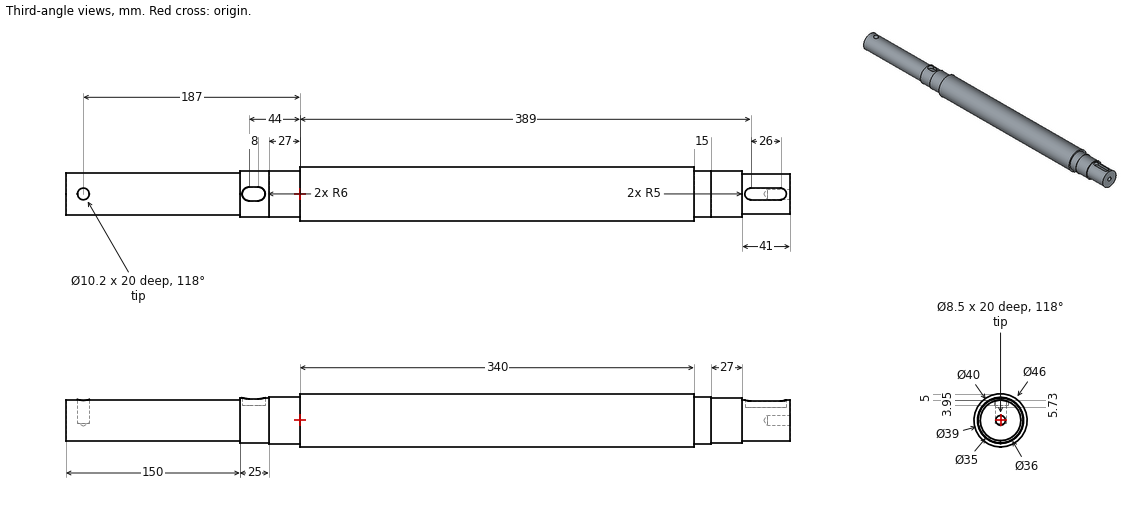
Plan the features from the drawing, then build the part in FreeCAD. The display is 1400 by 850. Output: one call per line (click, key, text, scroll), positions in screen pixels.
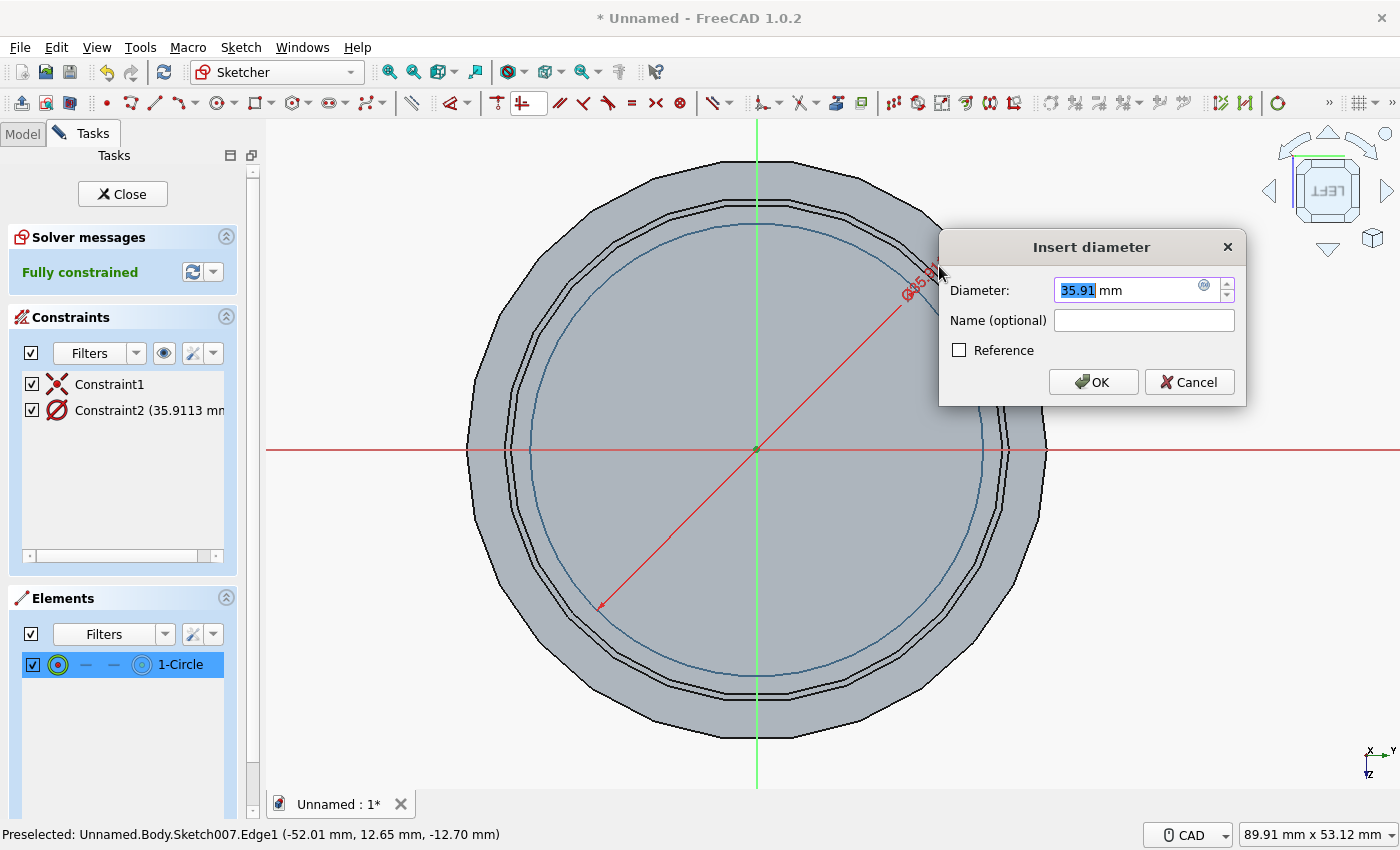
text(36)
key(Return)
key(Escape)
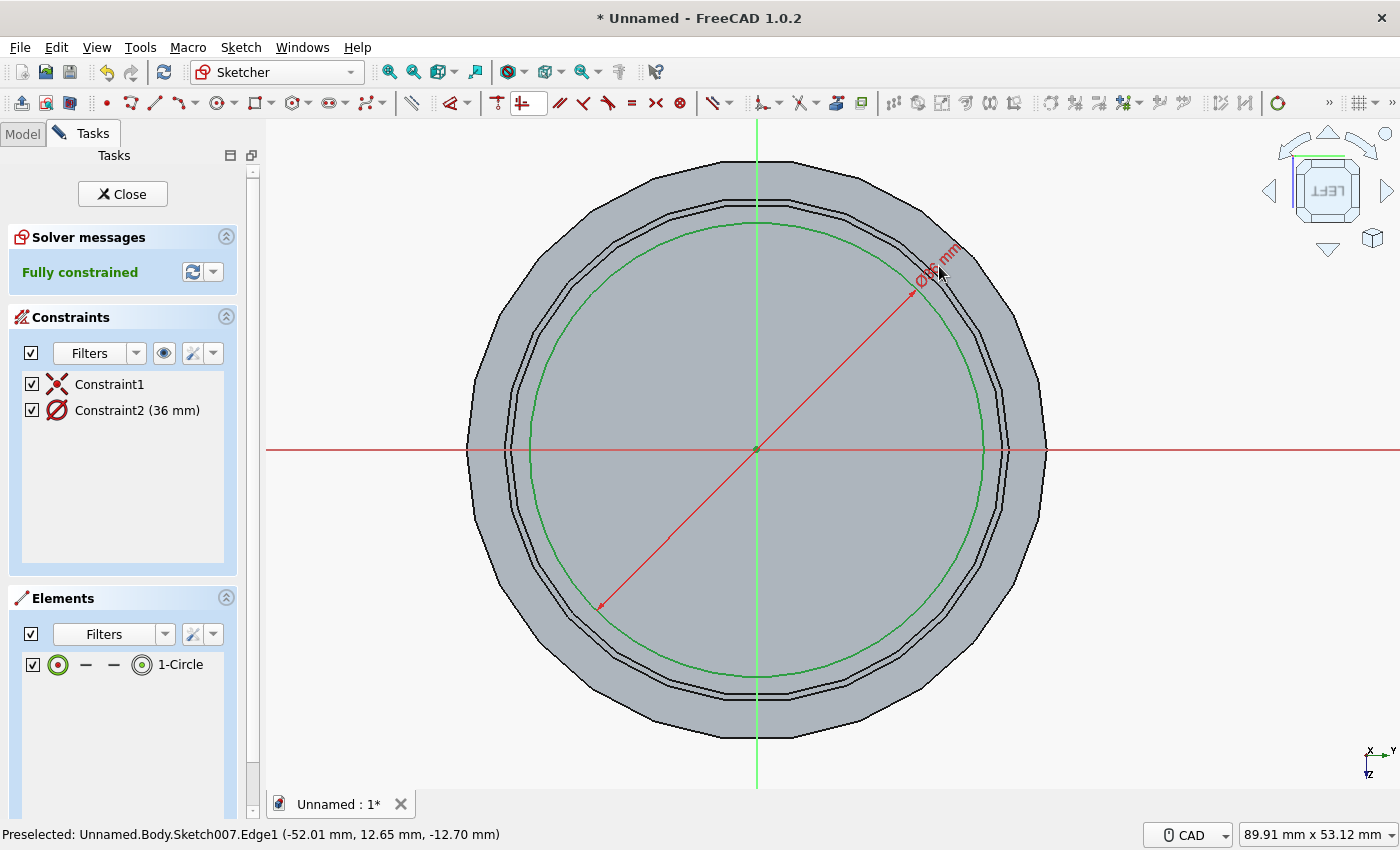
click(123, 194)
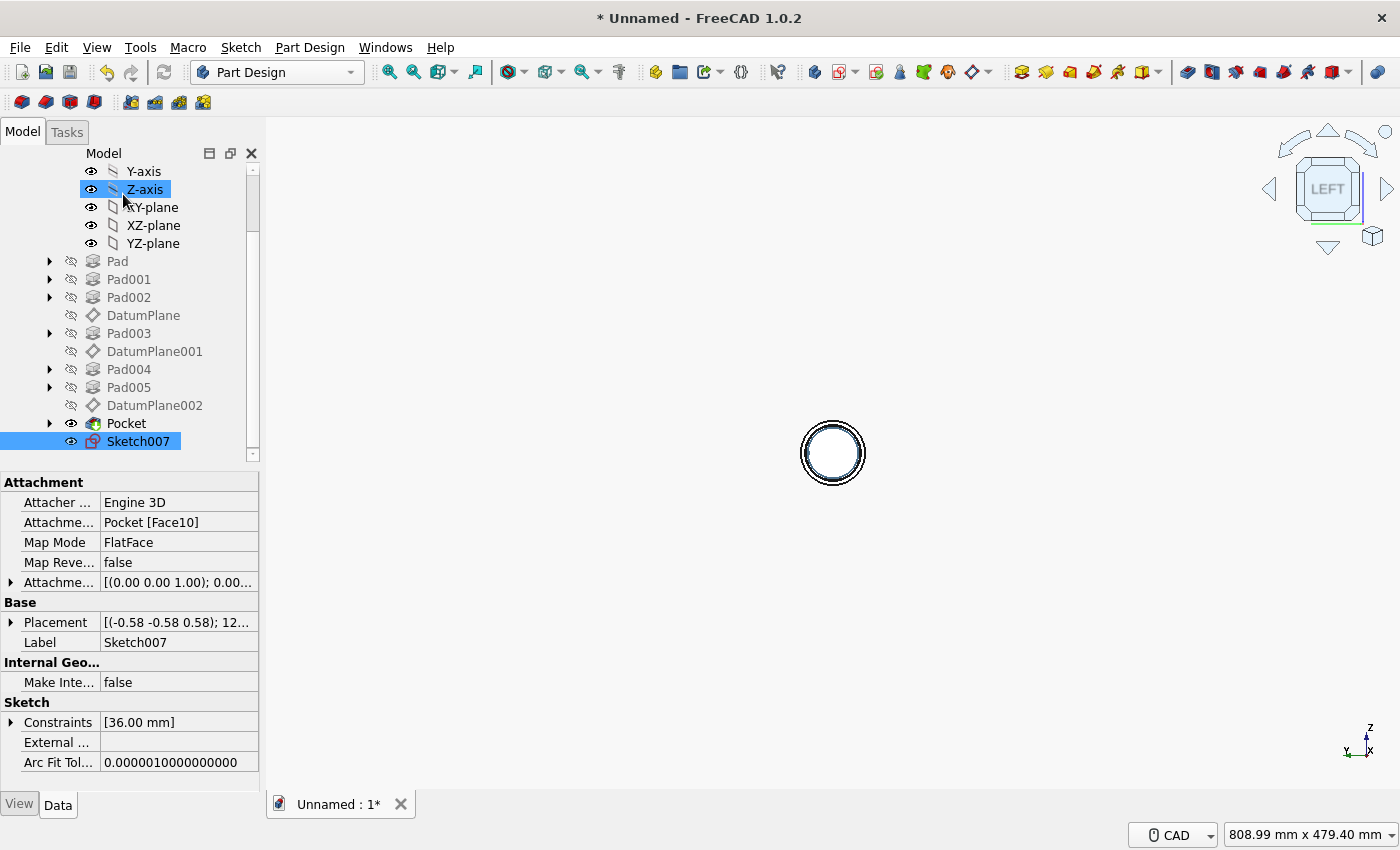
click(1022, 72)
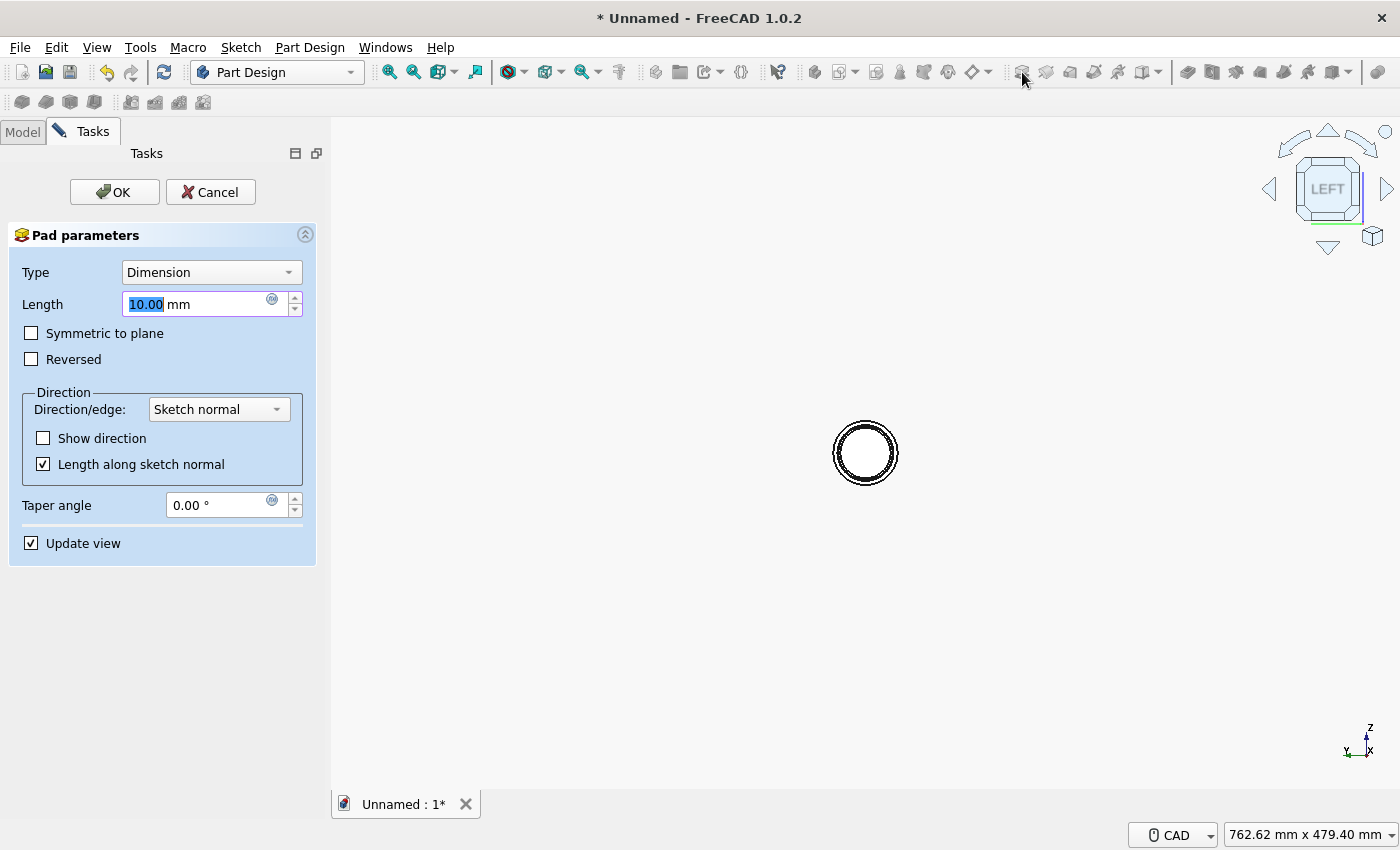
text(150)
key(Tab)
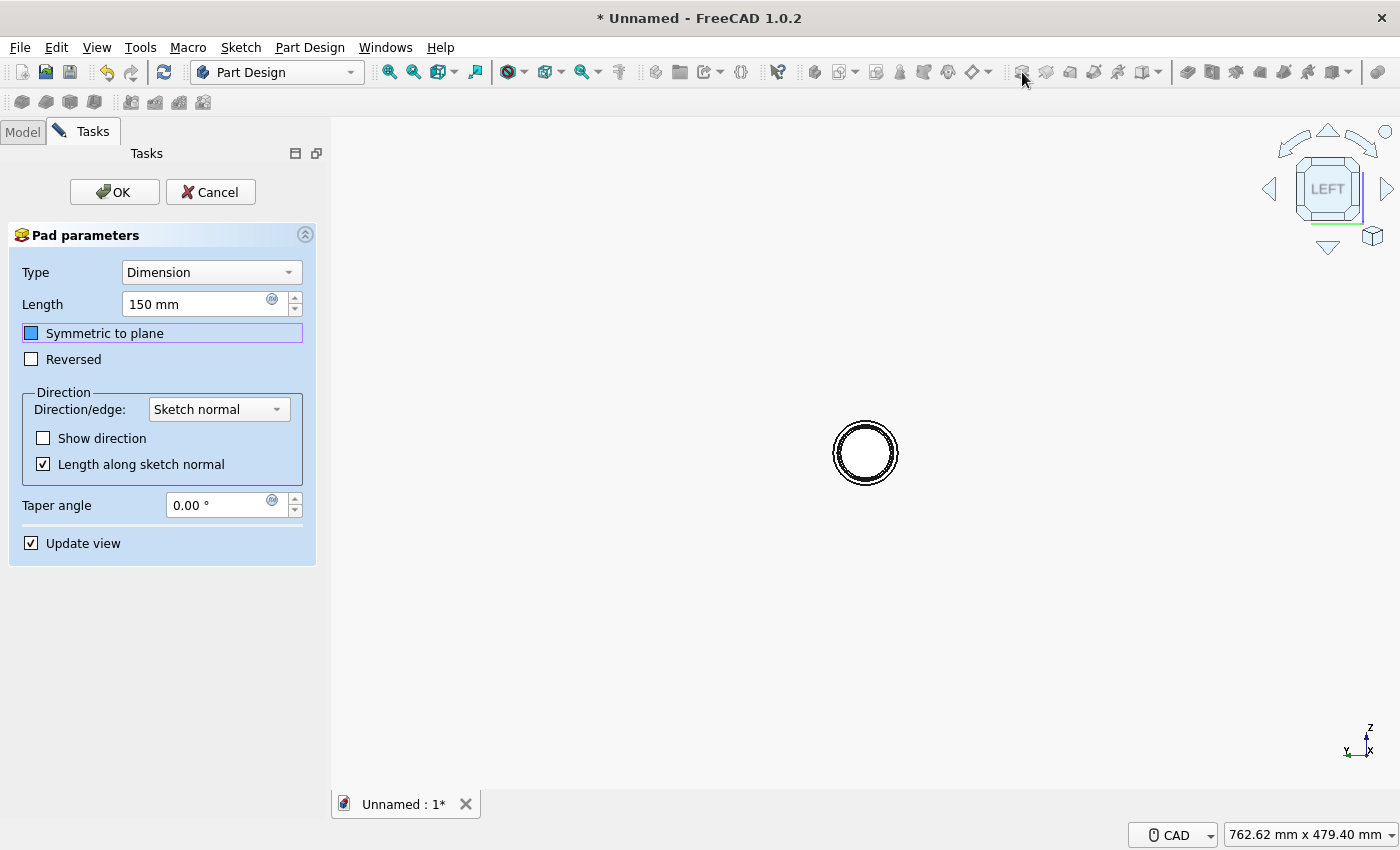
click(115, 192)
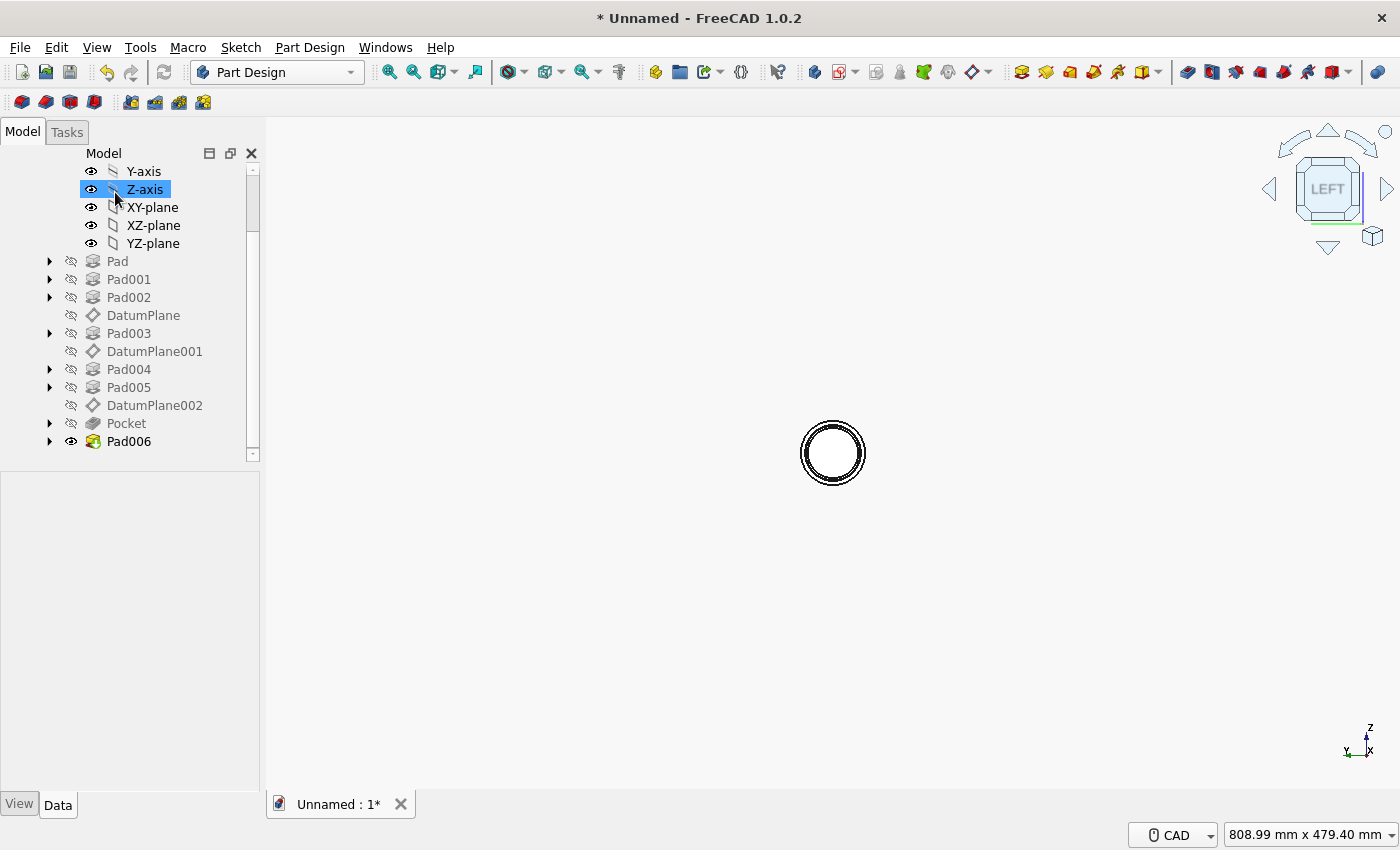
click(390, 72)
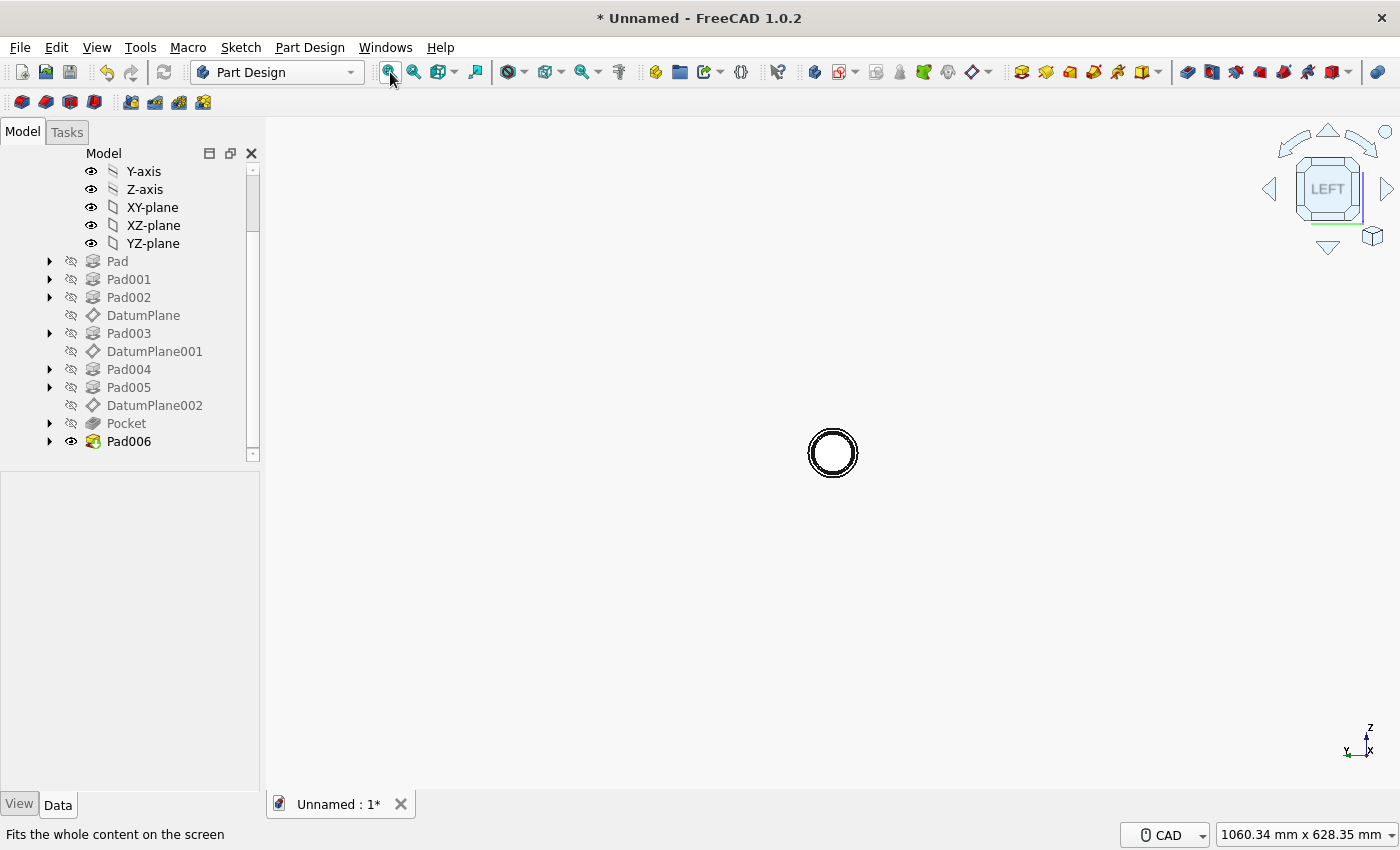
scroll(160, 311, down, 3)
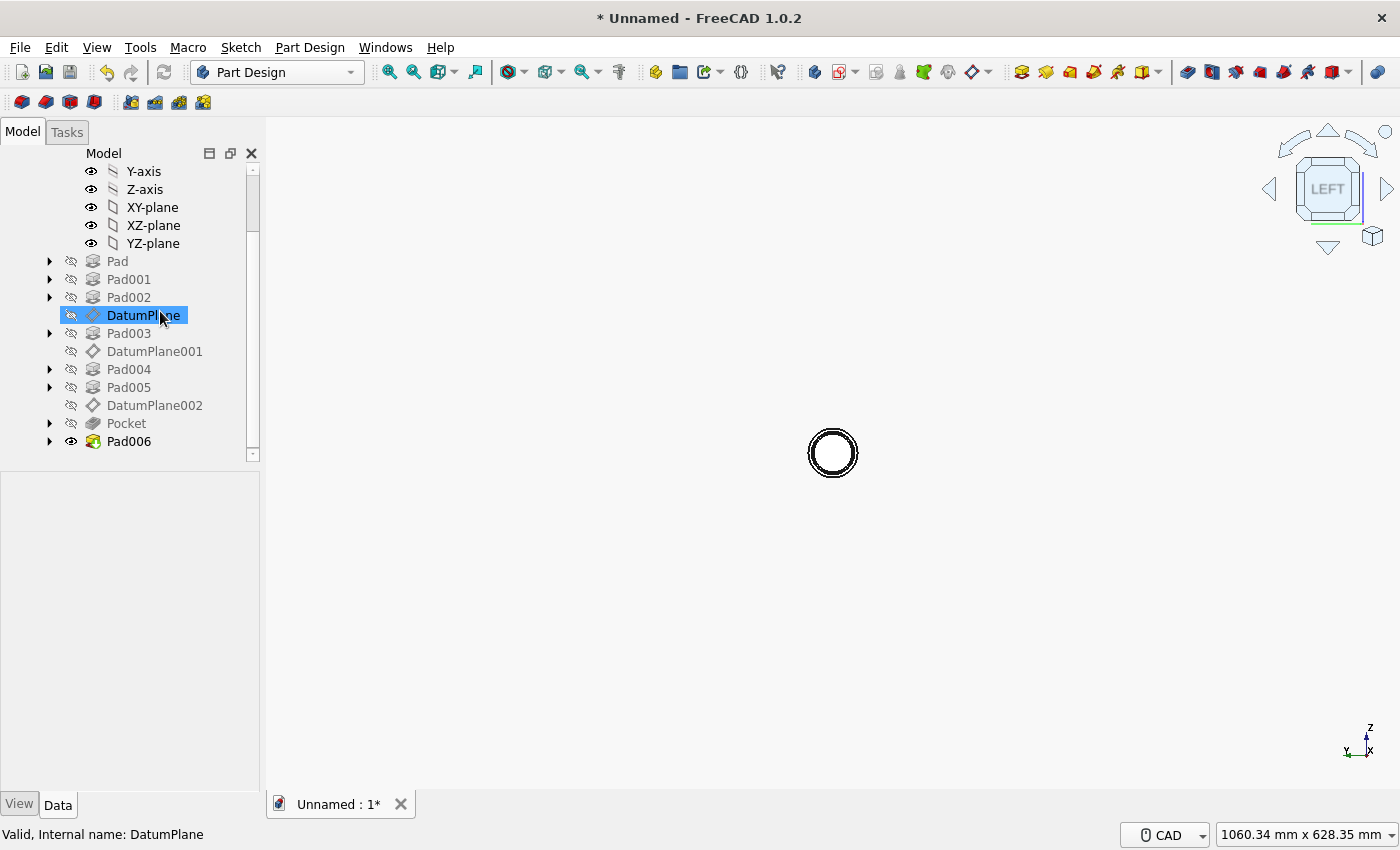
scroll(160, 311, up, 15)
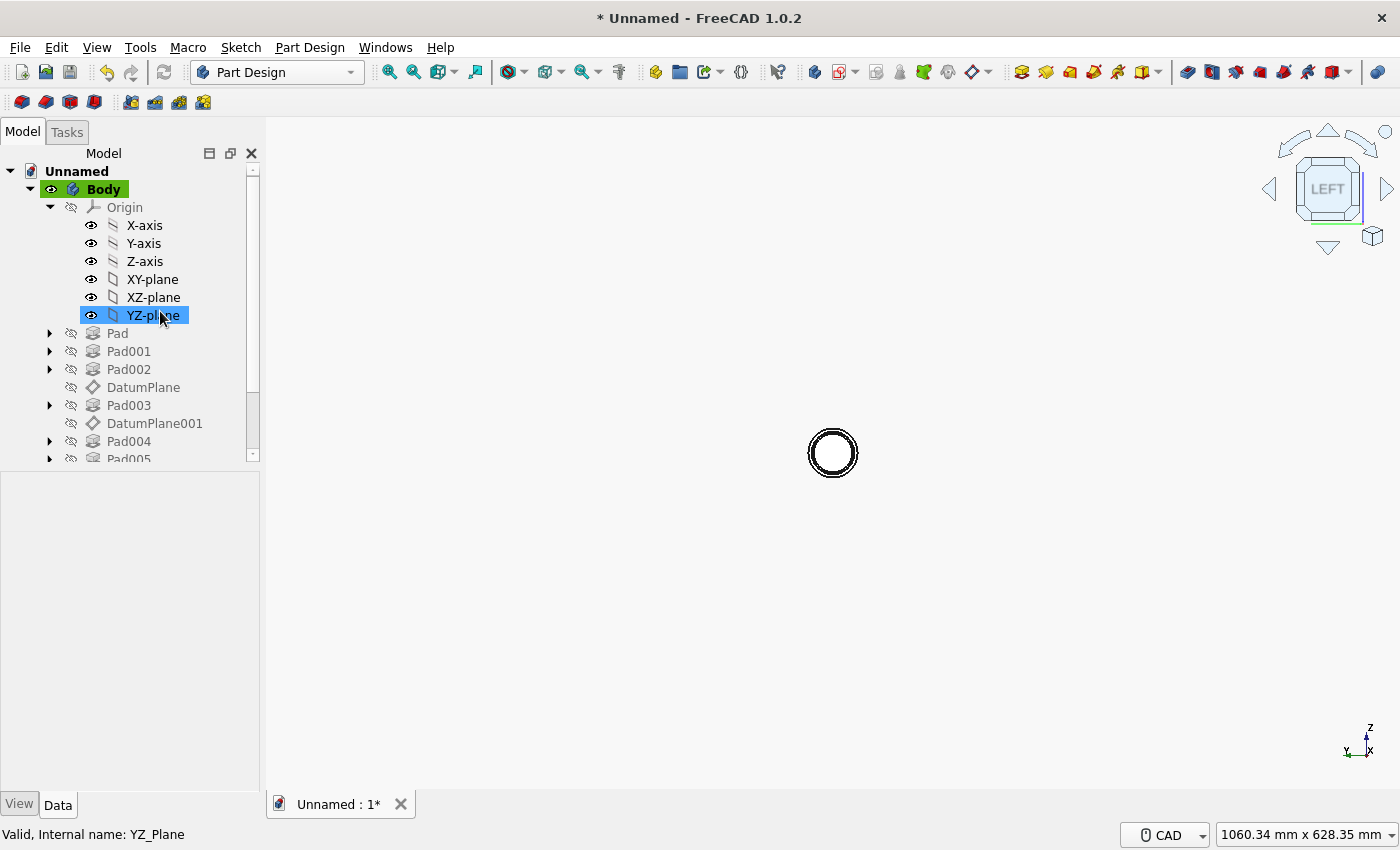
click(136, 279)